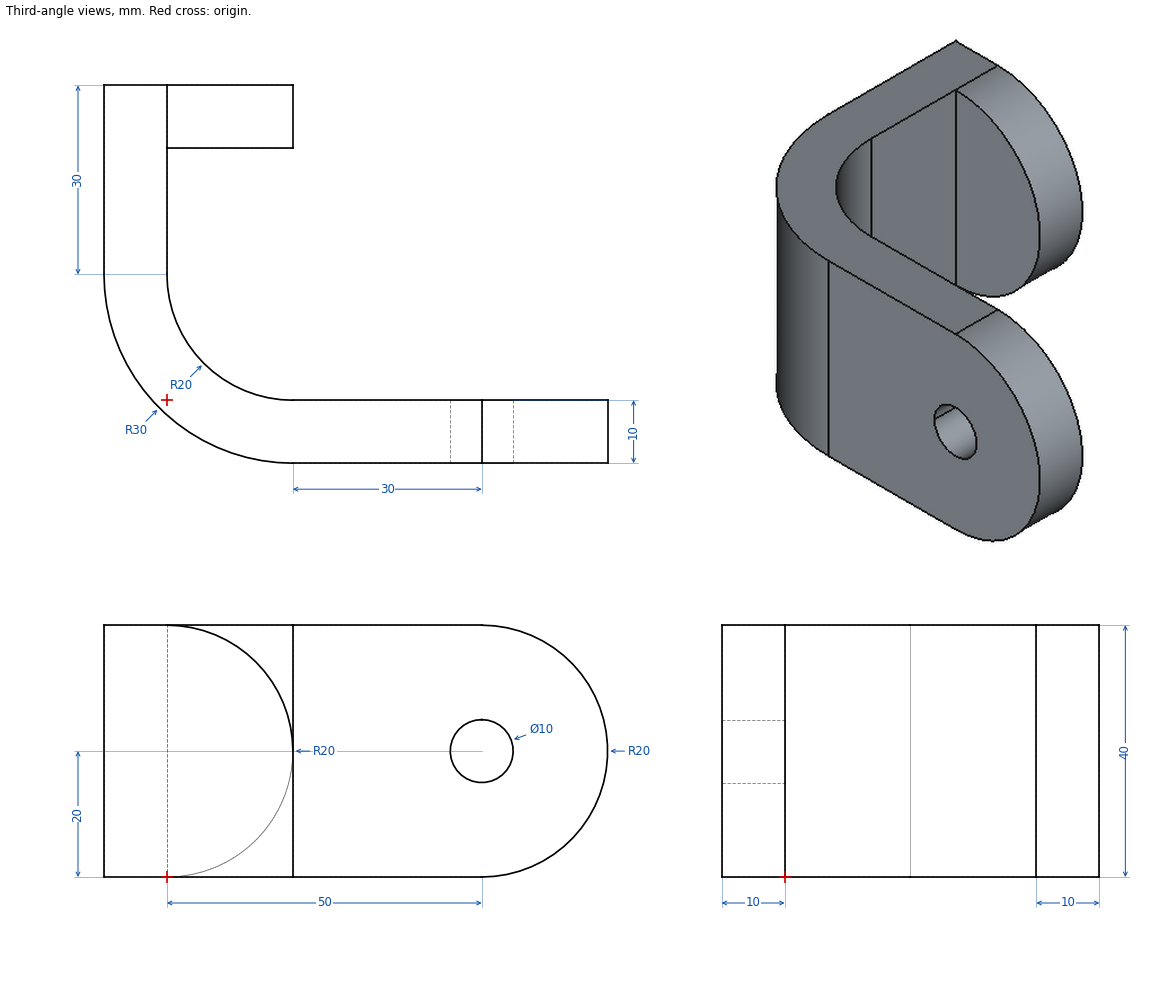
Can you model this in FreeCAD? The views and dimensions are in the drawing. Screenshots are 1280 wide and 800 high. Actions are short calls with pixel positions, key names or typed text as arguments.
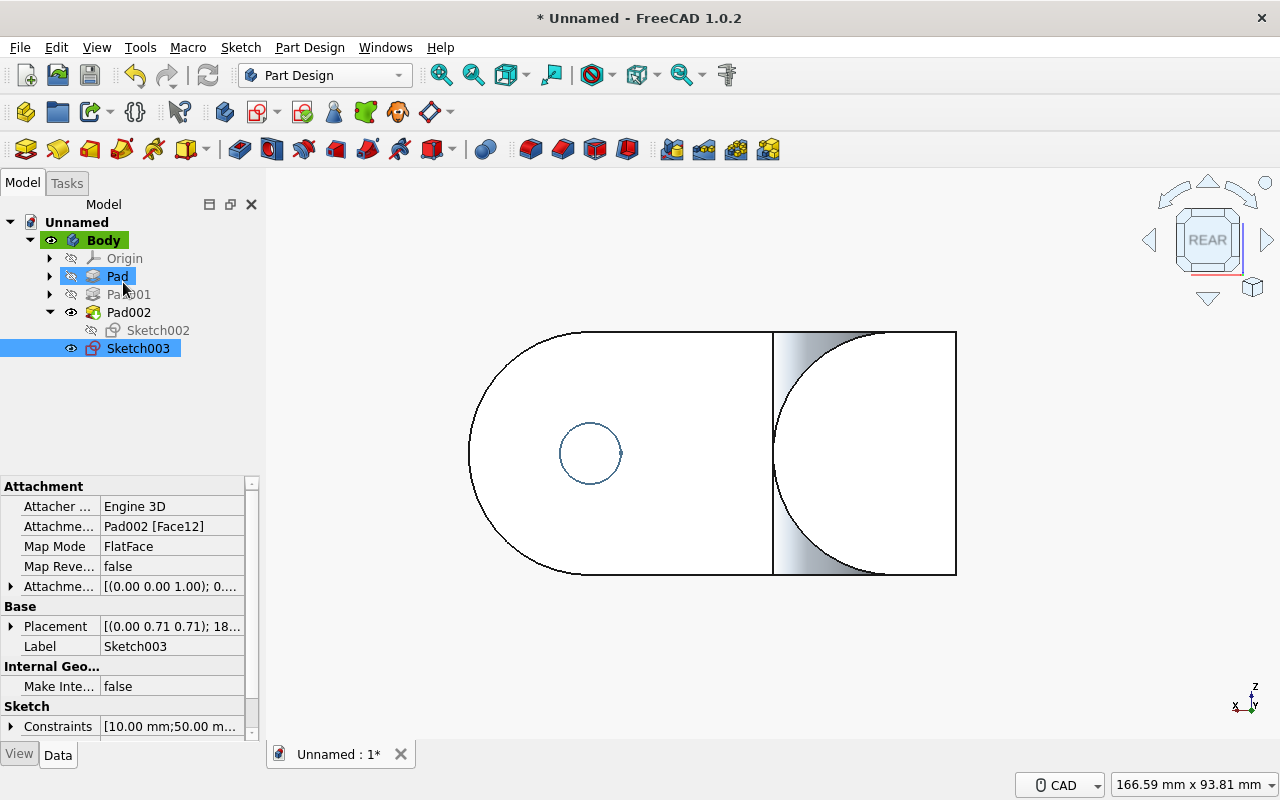
click(240, 150)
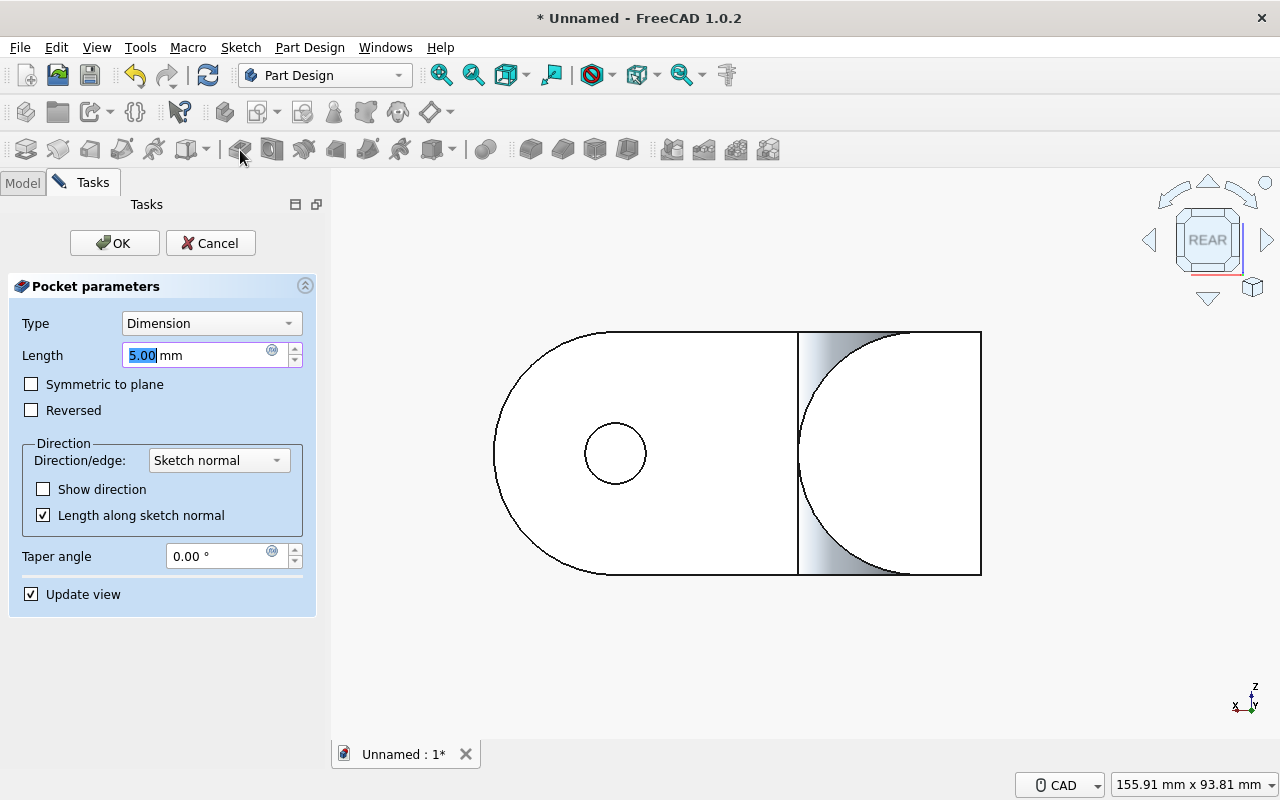
text(10)
key(Tab)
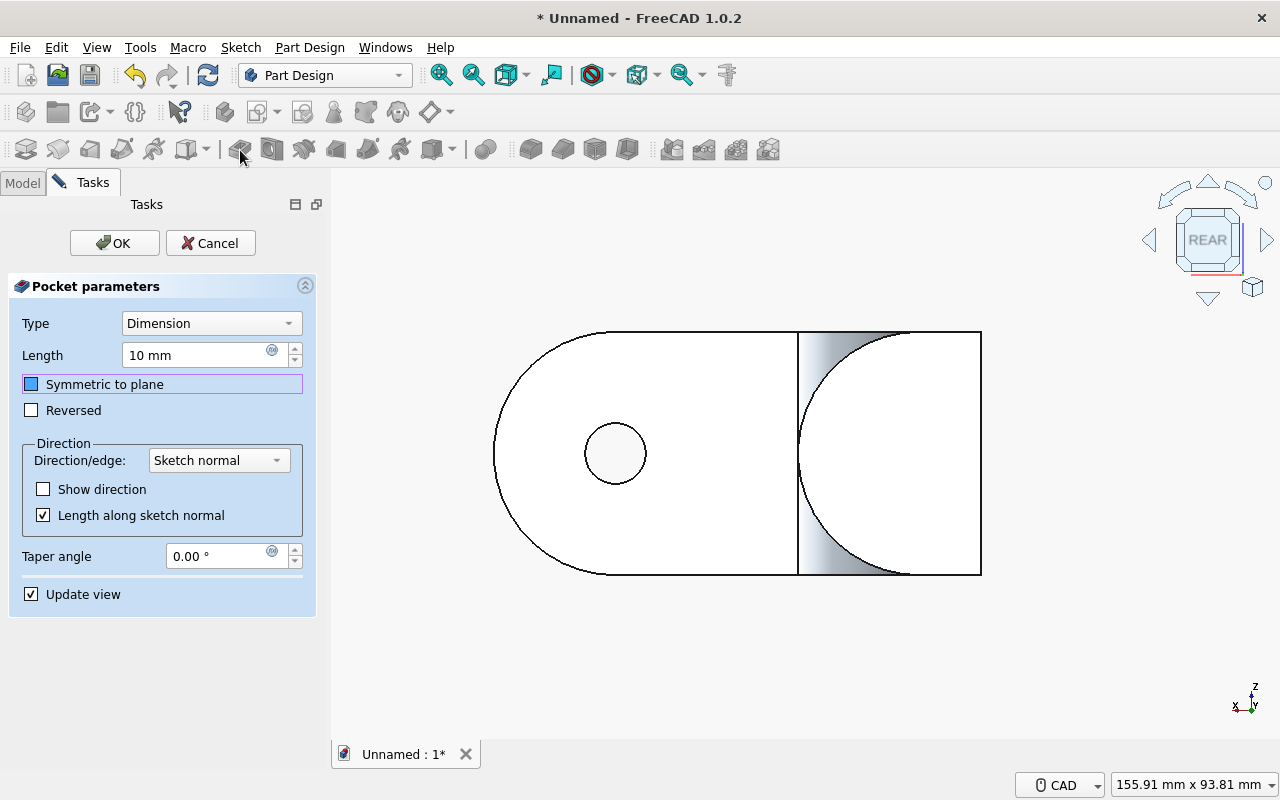
click(115, 243)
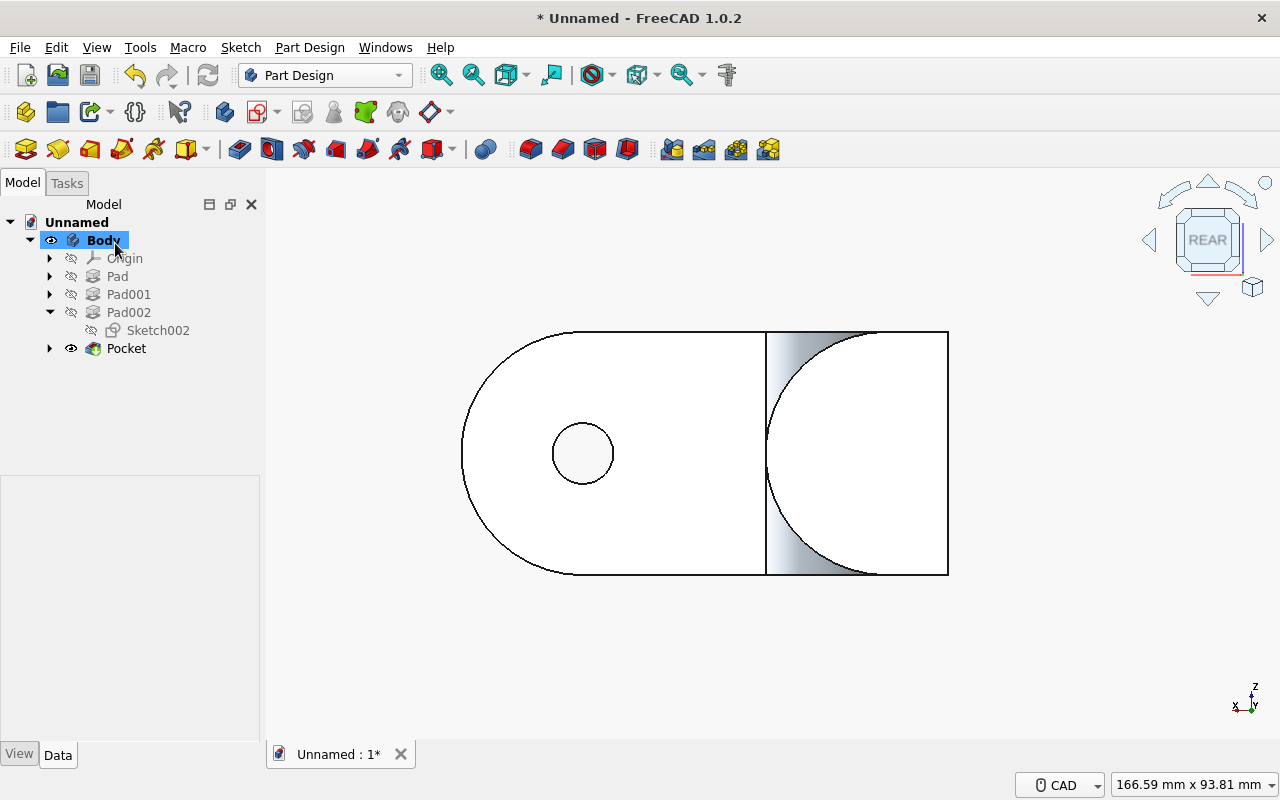
key(0)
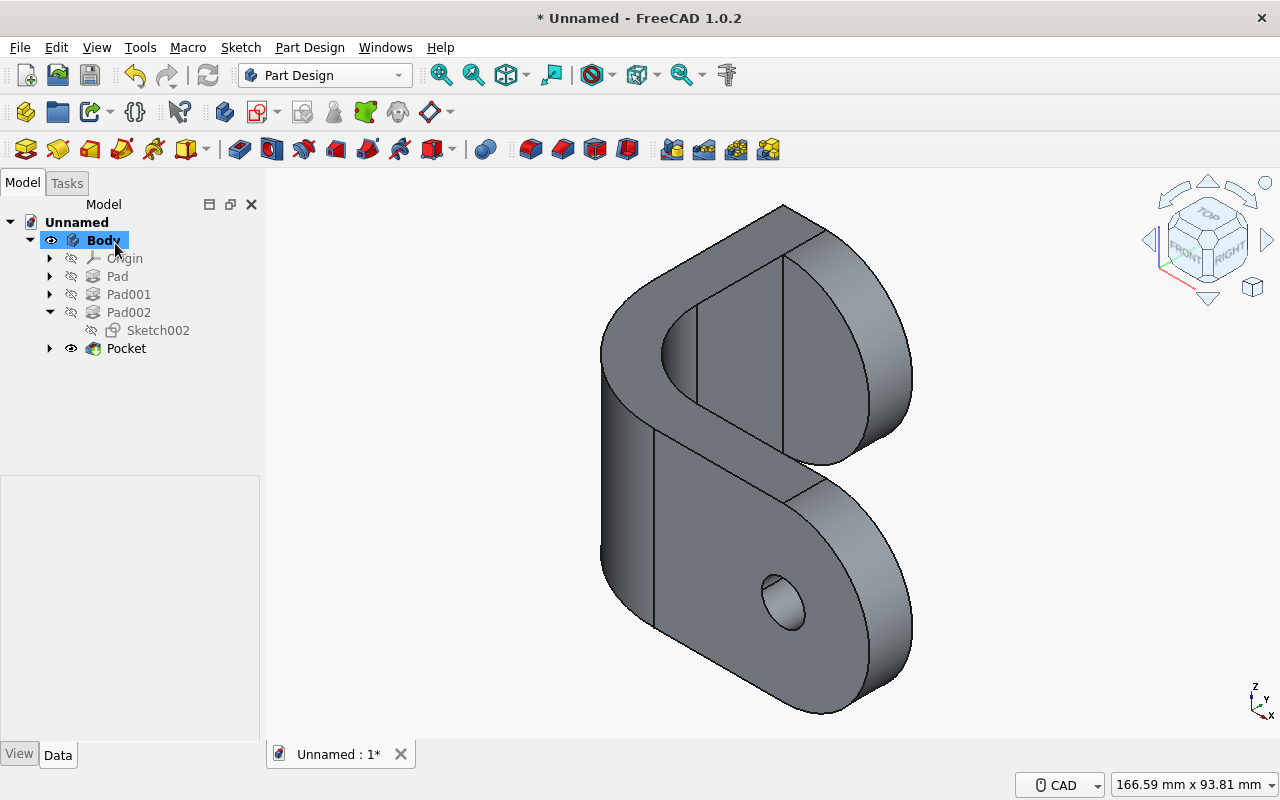
click(442, 76)